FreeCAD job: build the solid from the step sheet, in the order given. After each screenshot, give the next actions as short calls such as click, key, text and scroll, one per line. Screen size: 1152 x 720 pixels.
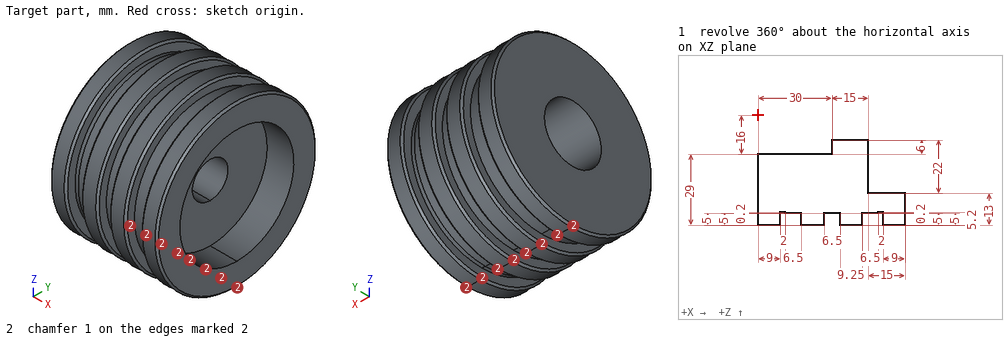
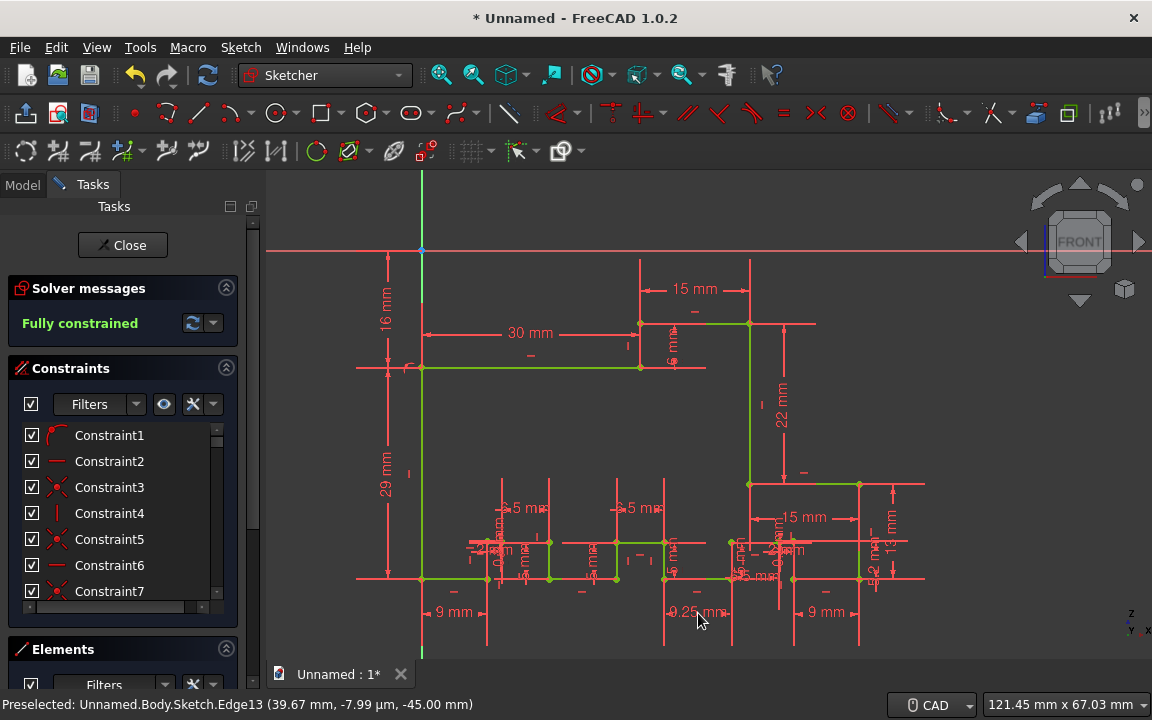
click(123, 245)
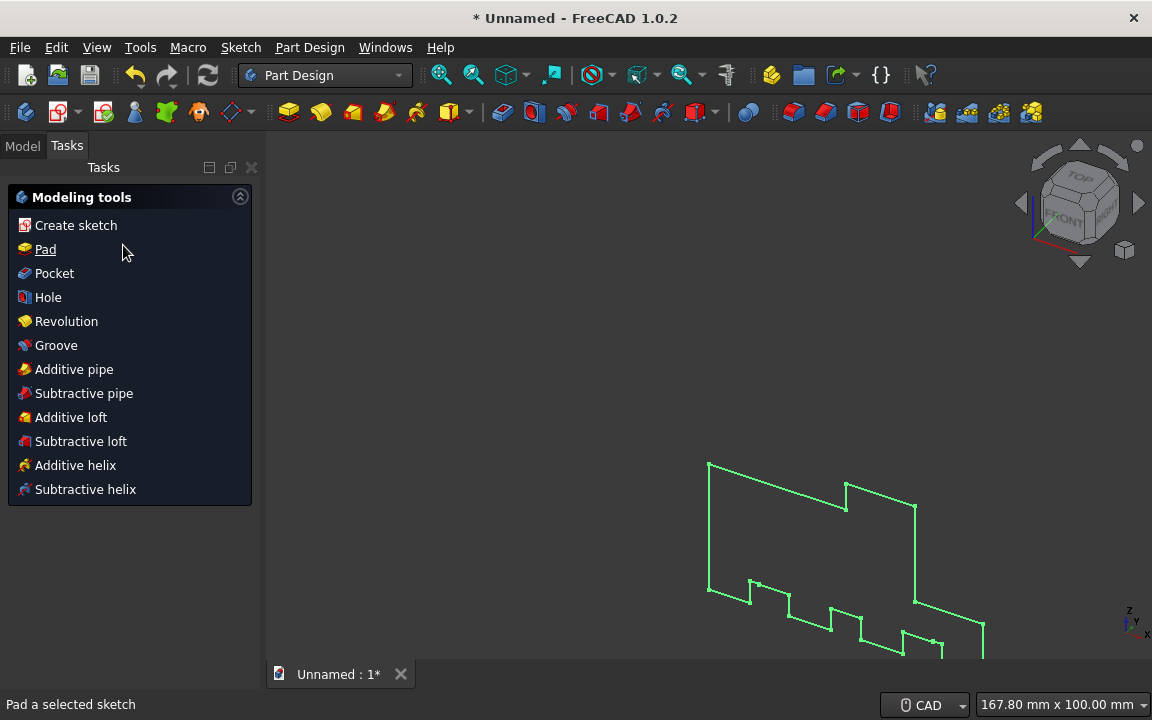
click(322, 112)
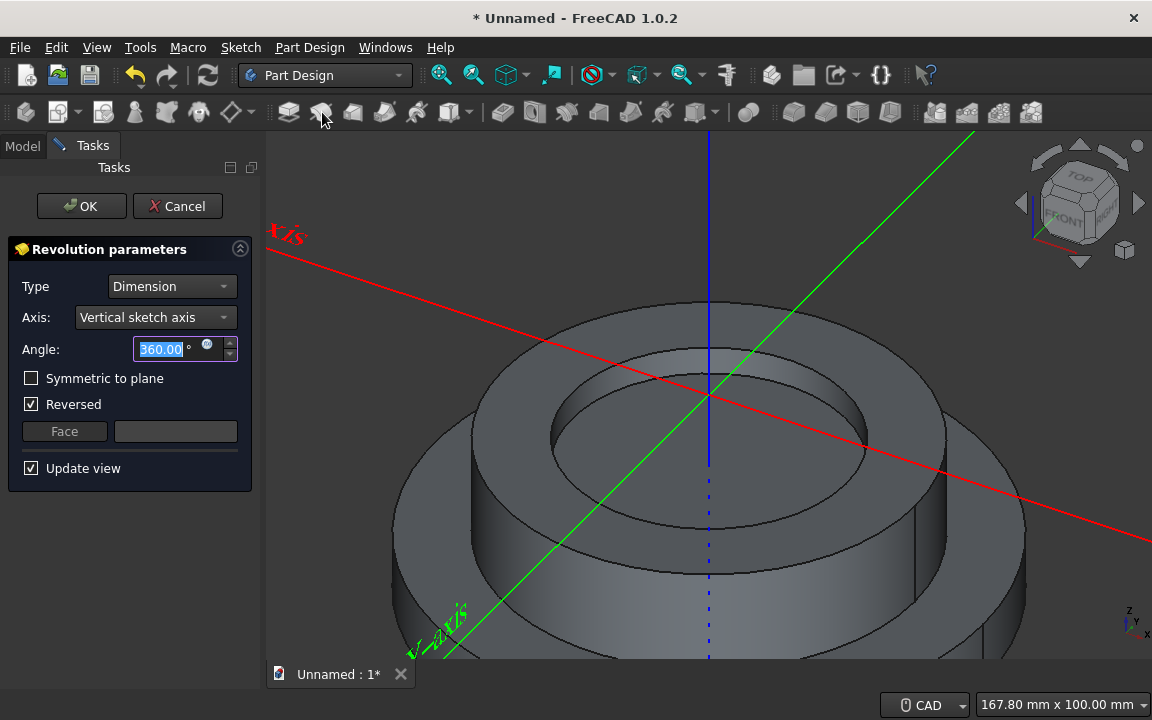
click(156, 318)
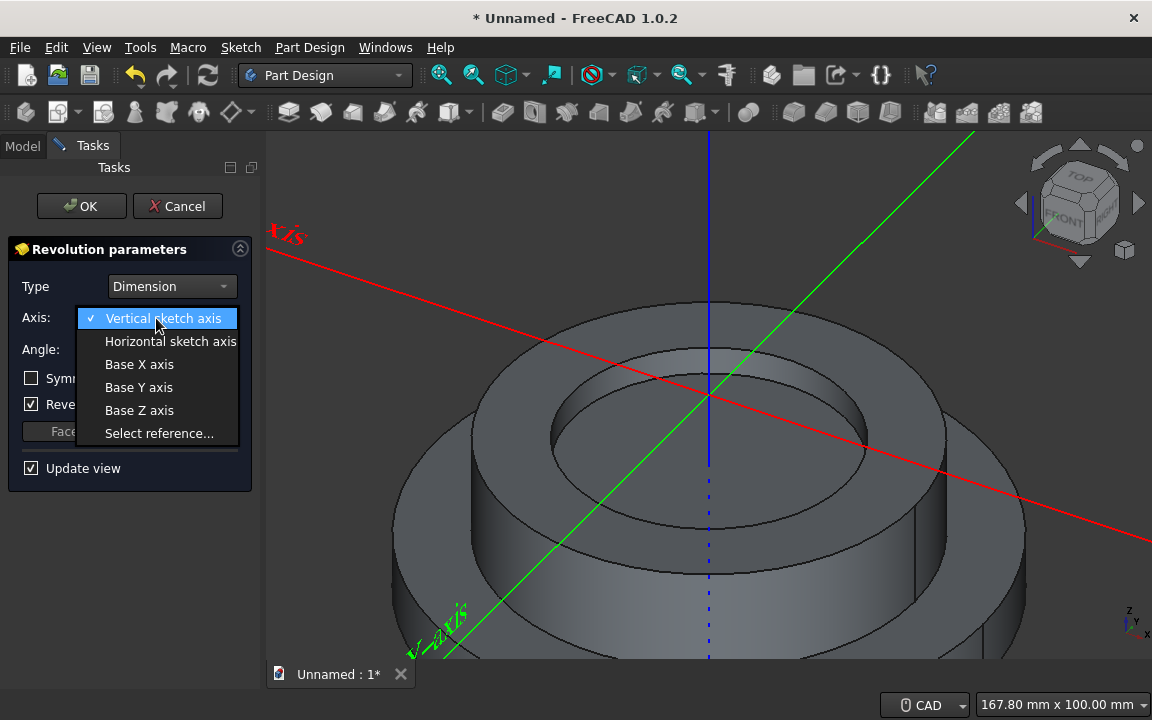
click(156, 342)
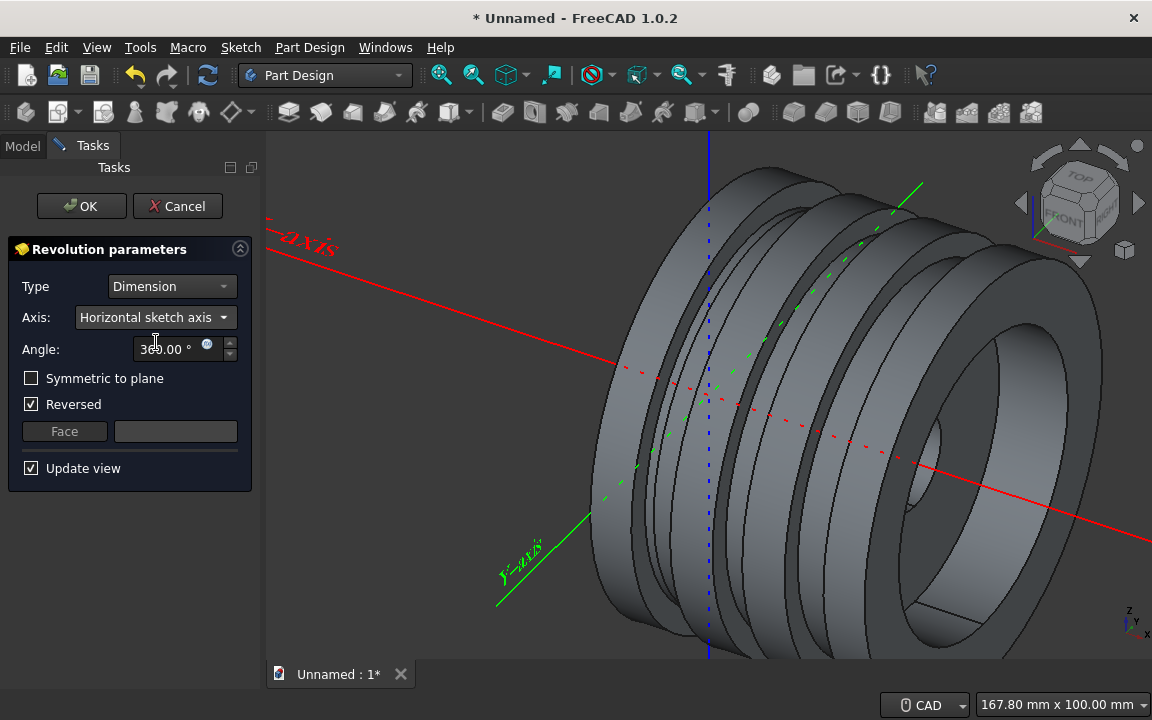
click(82, 206)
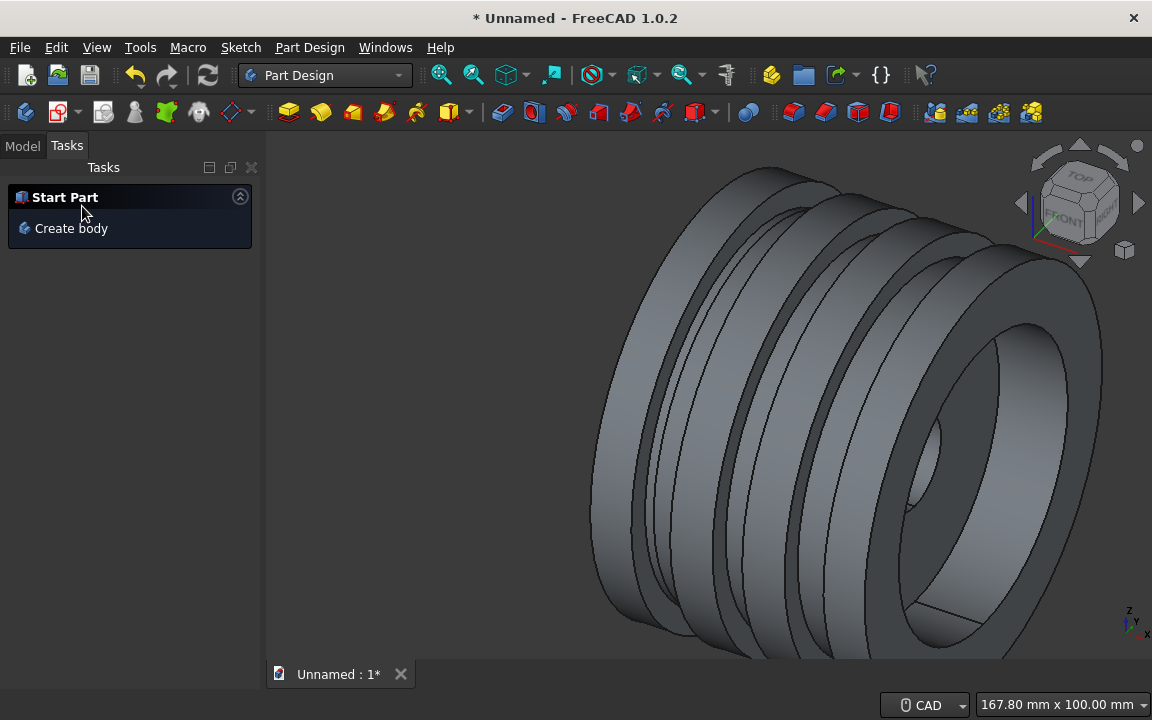
click(442, 76)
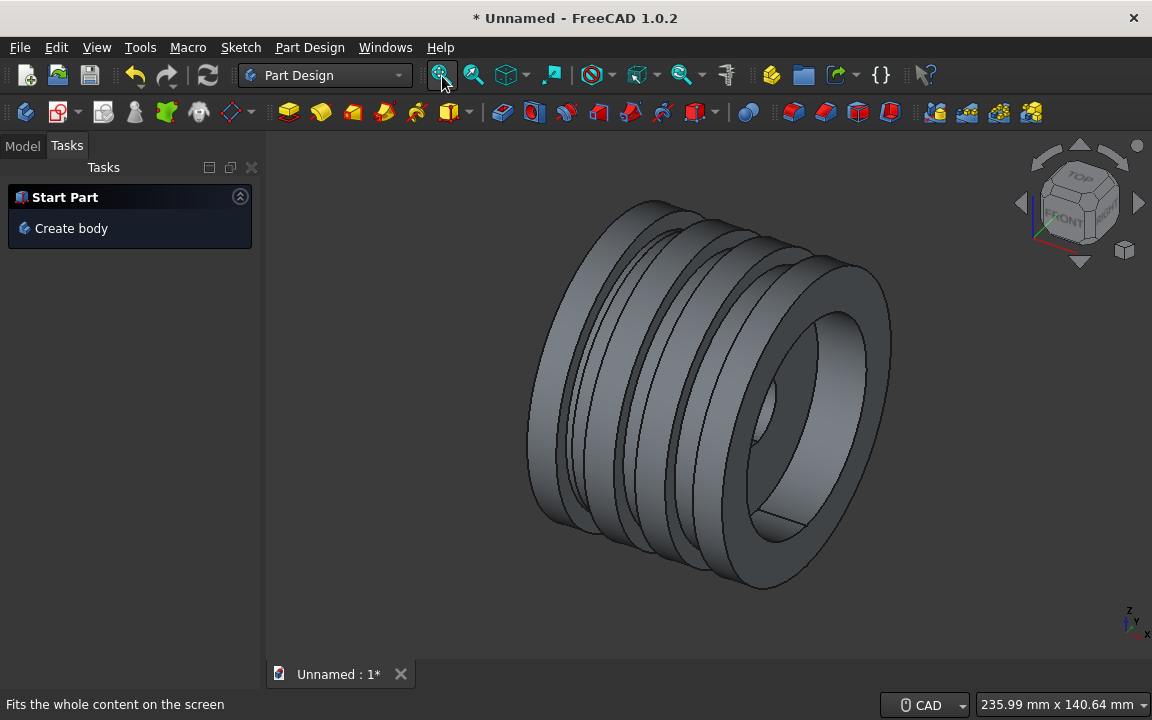
click(807, 288)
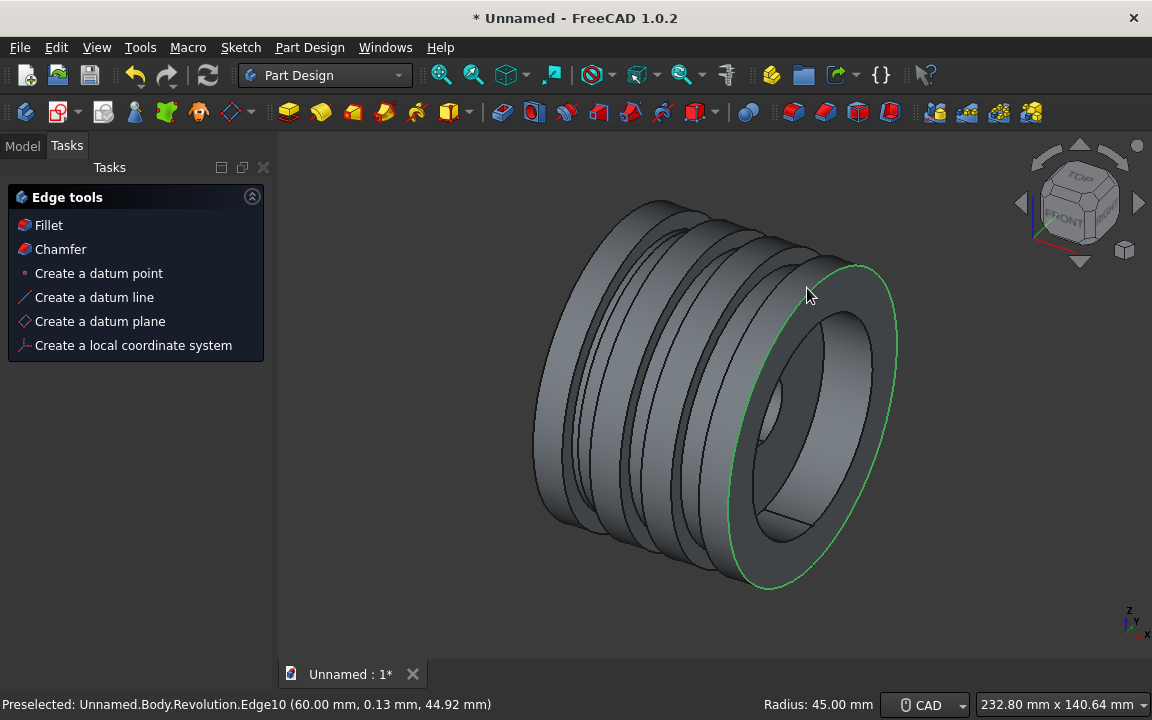
click(756, 269, ctrl)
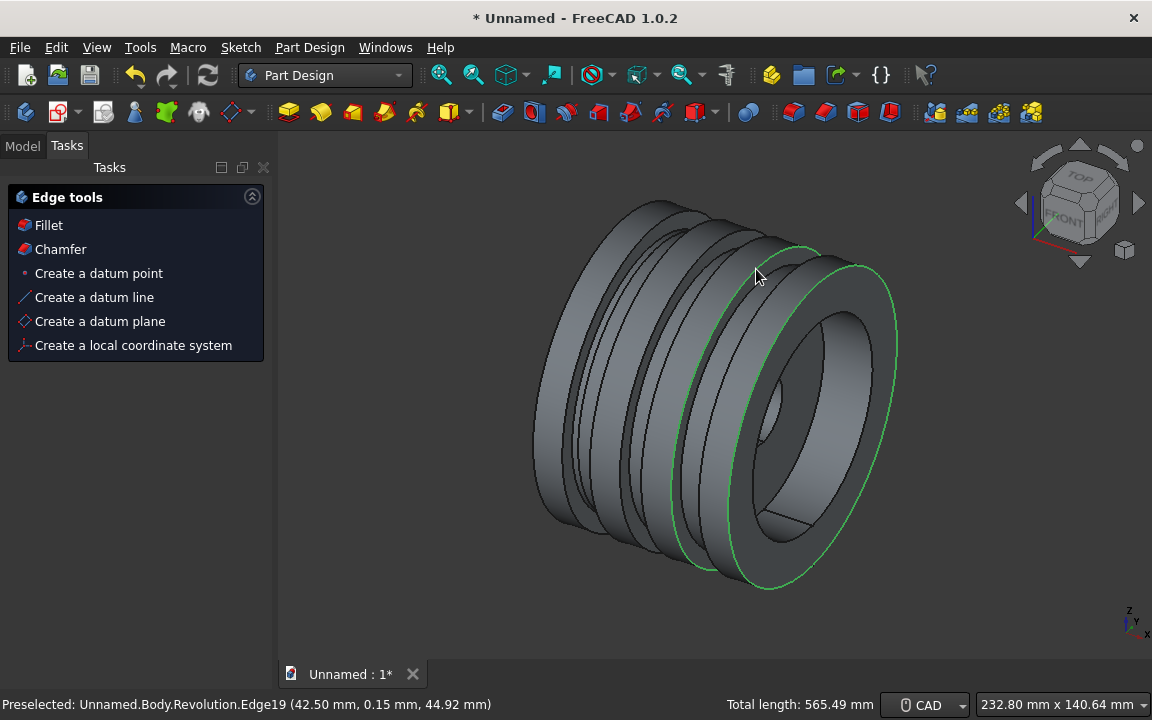
click(704, 252, ctrl)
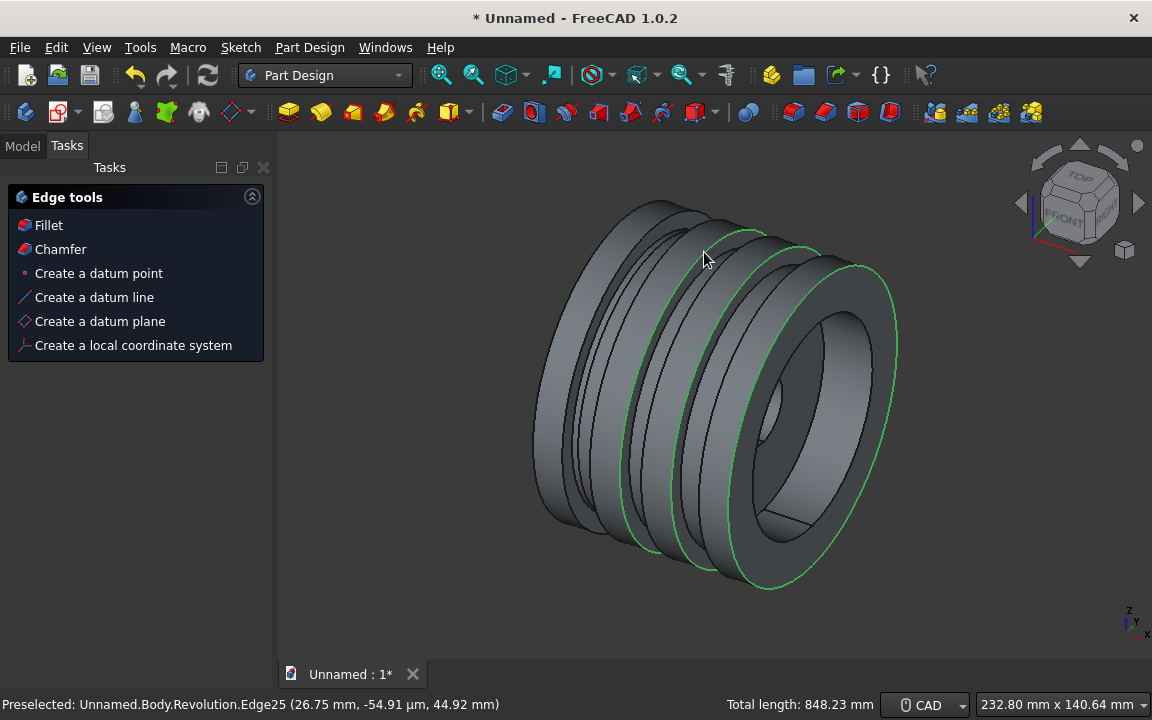
click(647, 233, ctrl)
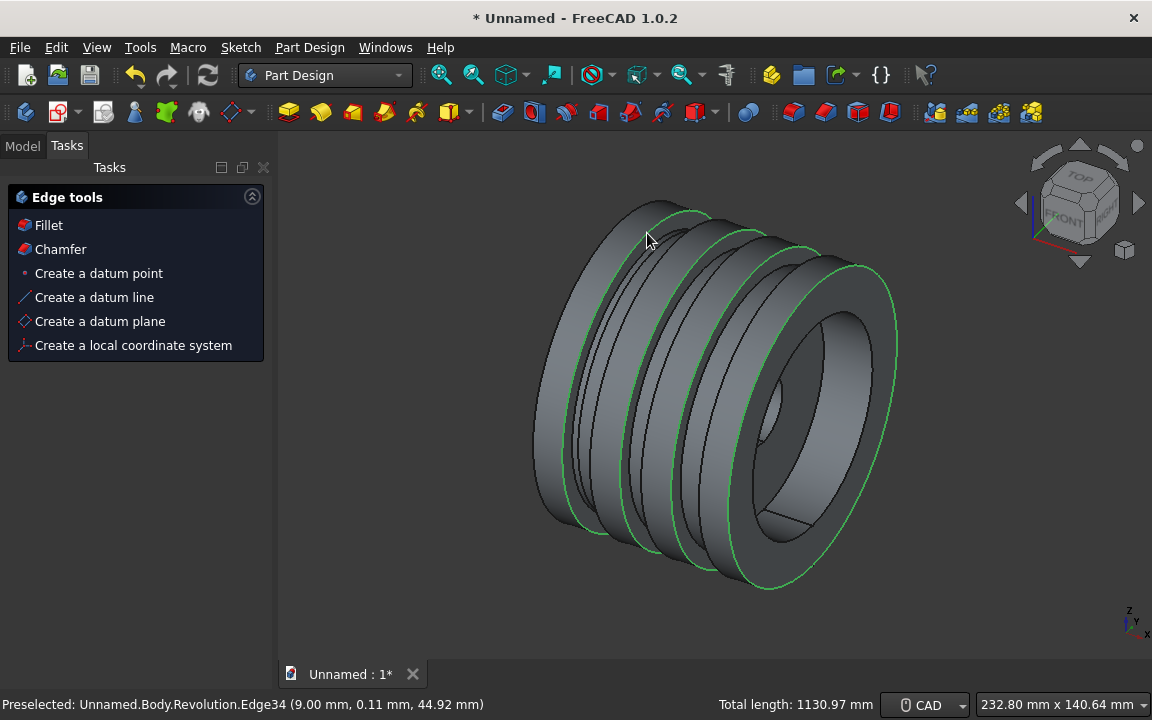
click(537, 399, ctrl)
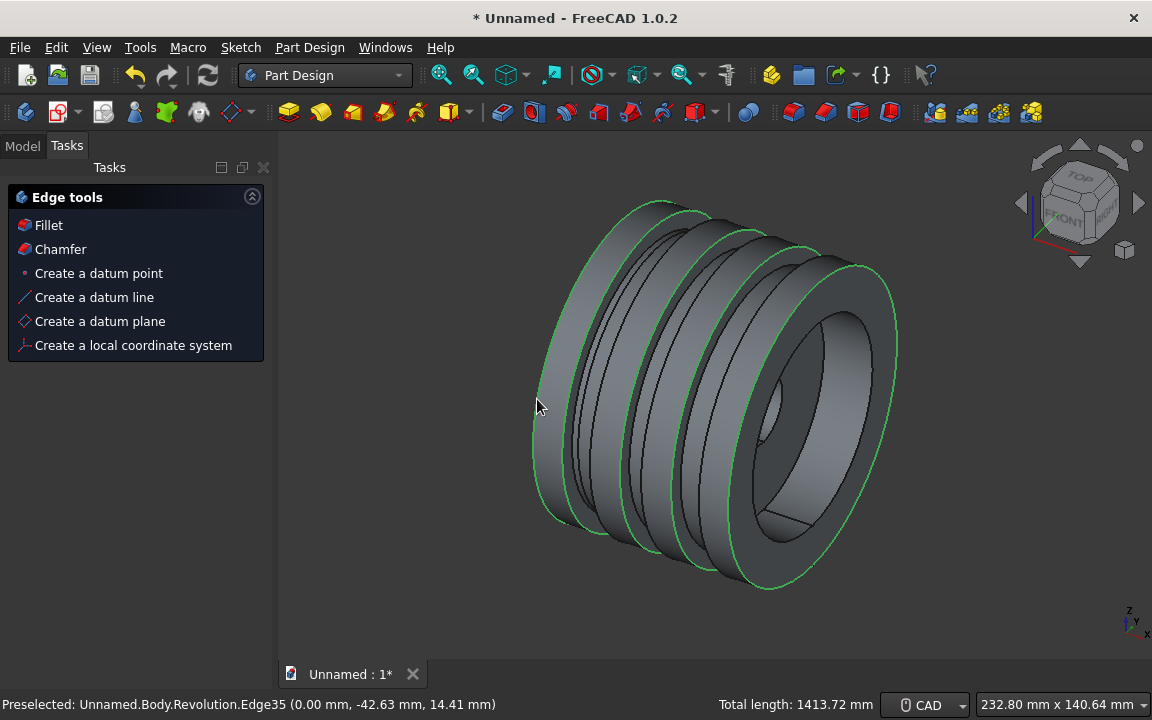
key(0)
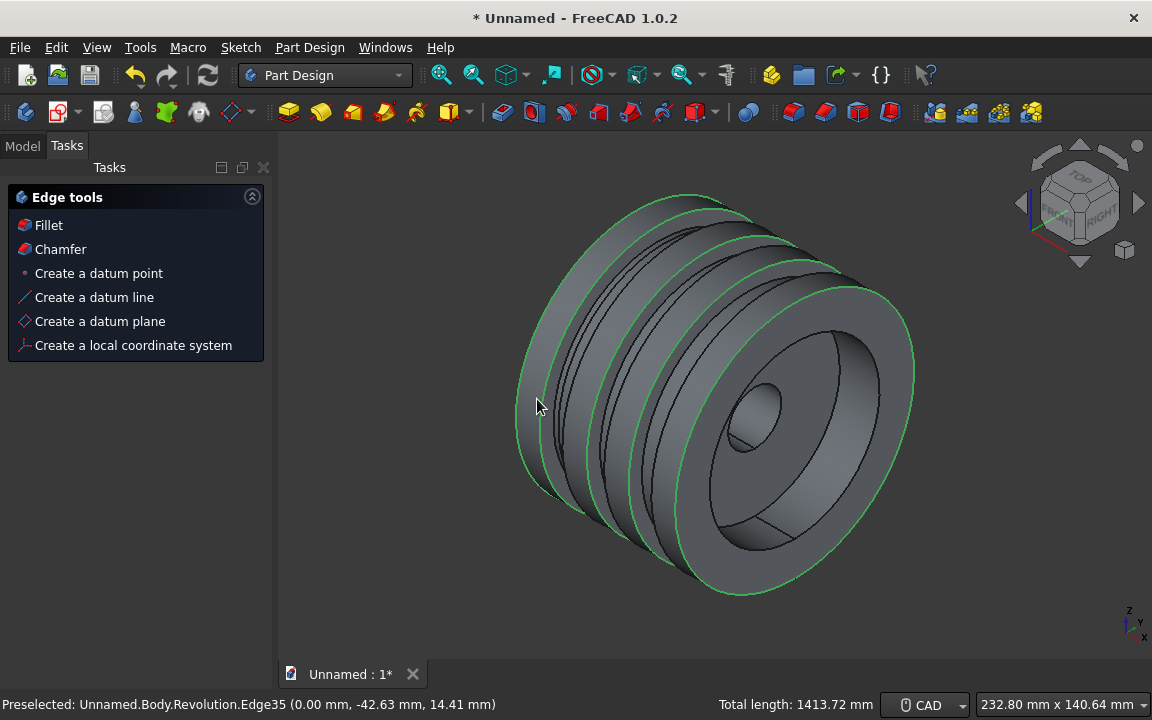
key(2)